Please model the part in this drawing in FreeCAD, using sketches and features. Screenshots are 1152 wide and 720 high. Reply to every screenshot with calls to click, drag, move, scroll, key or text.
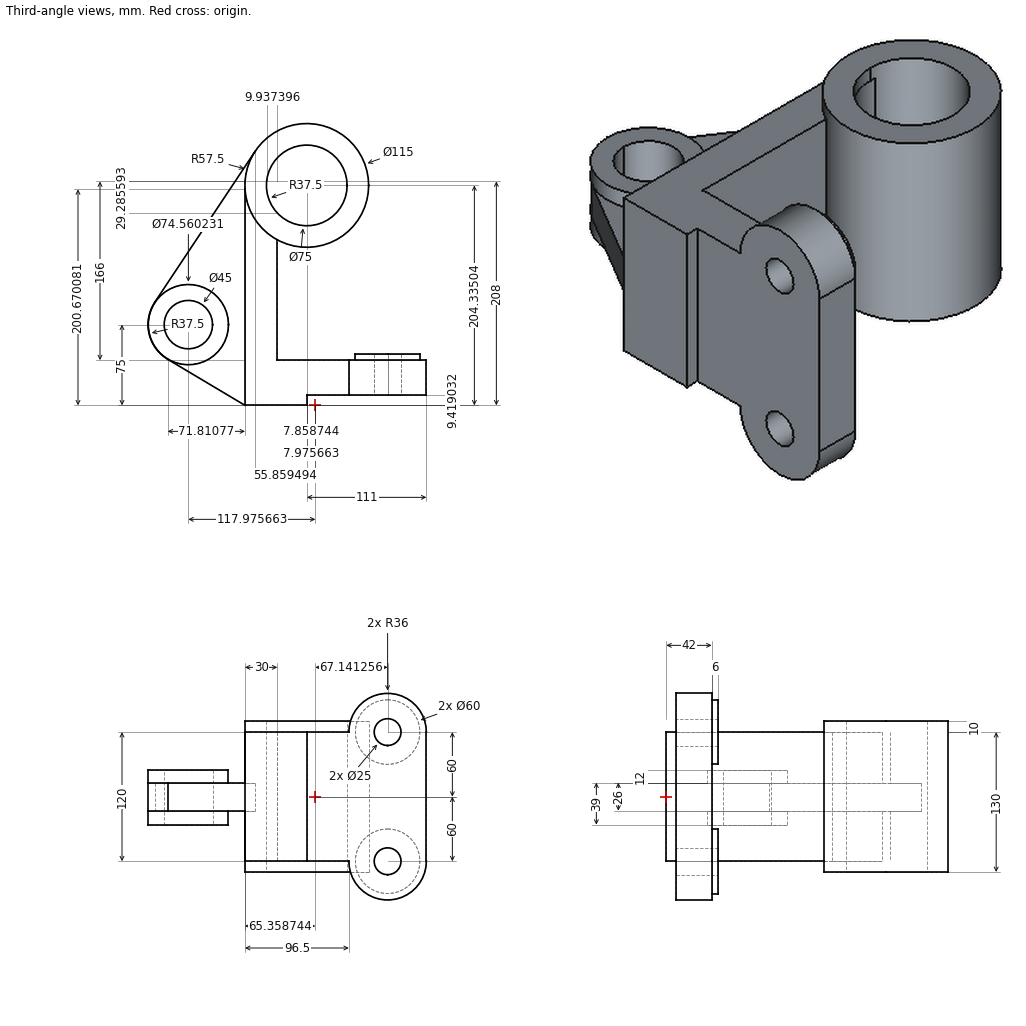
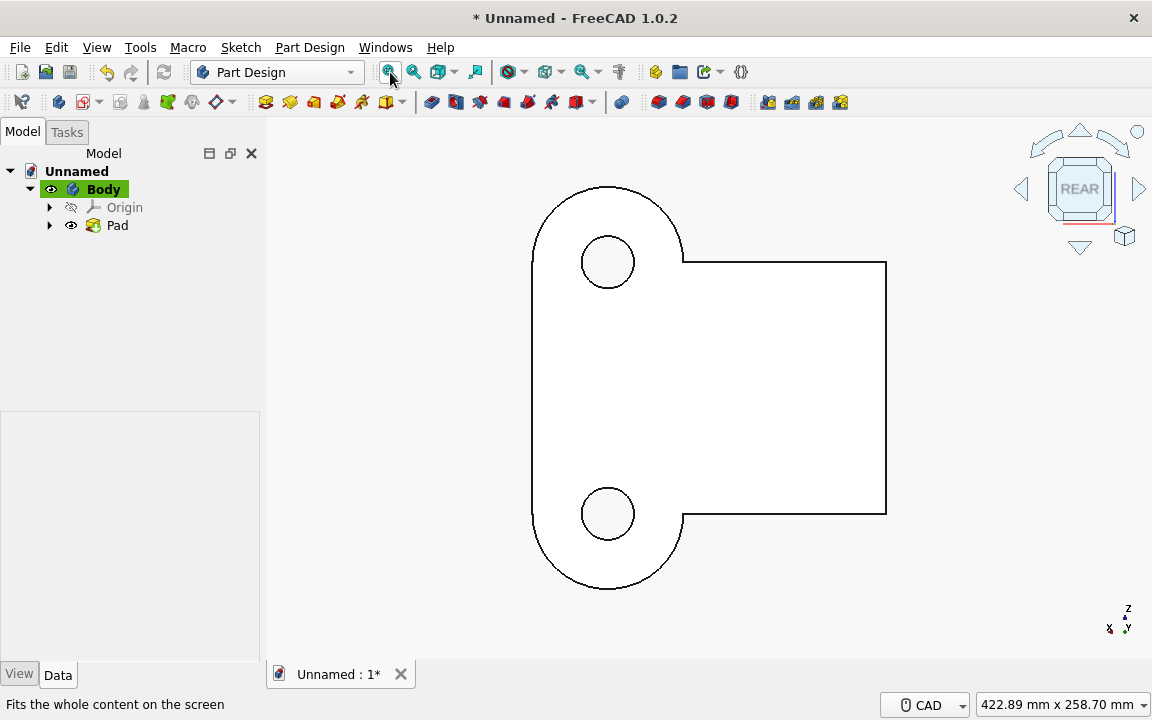
click(709, 387)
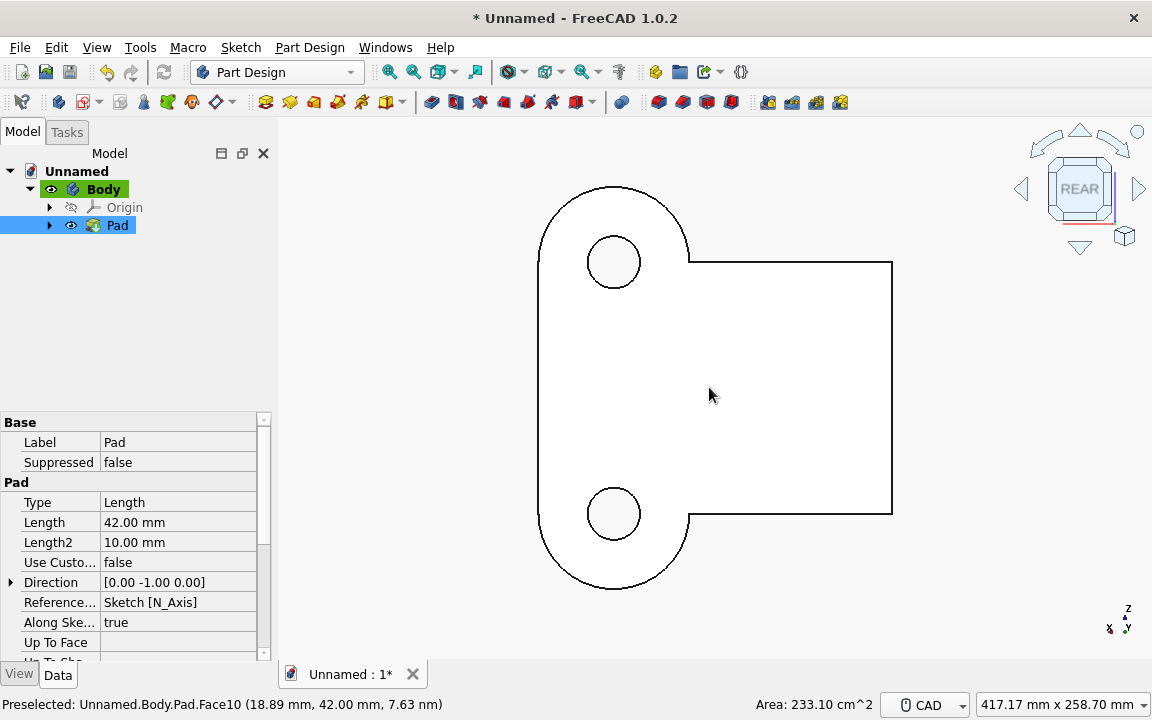
click(84, 102)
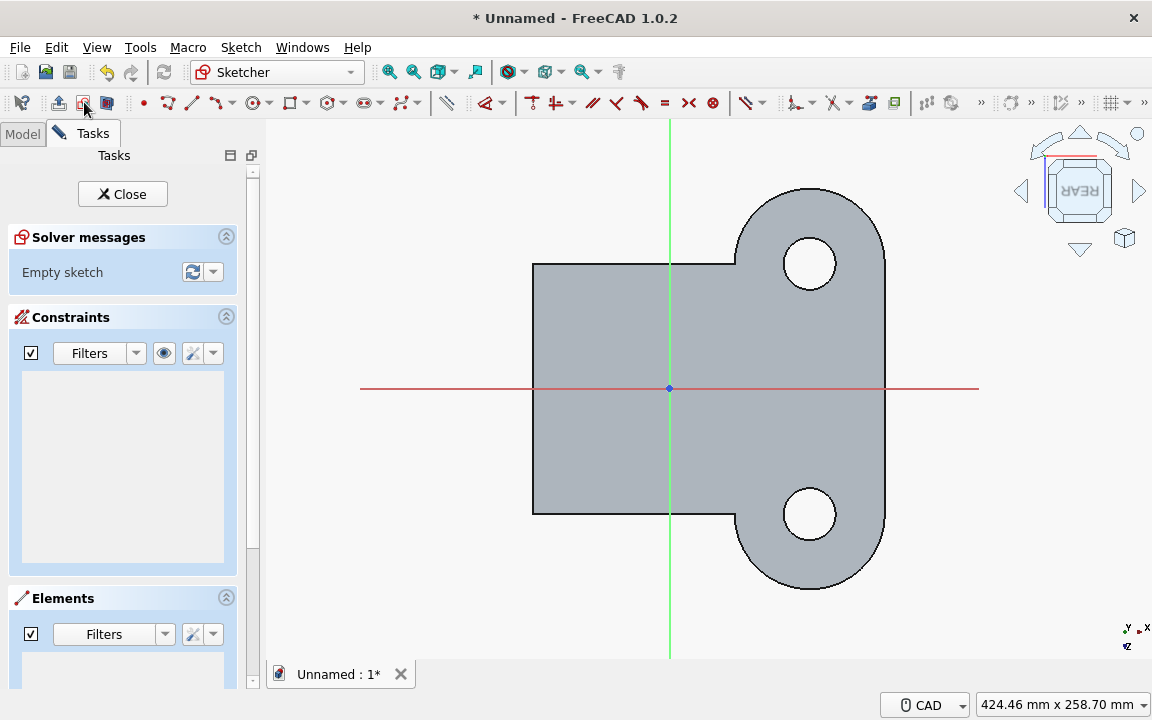
scroll(522, 389, up, 2)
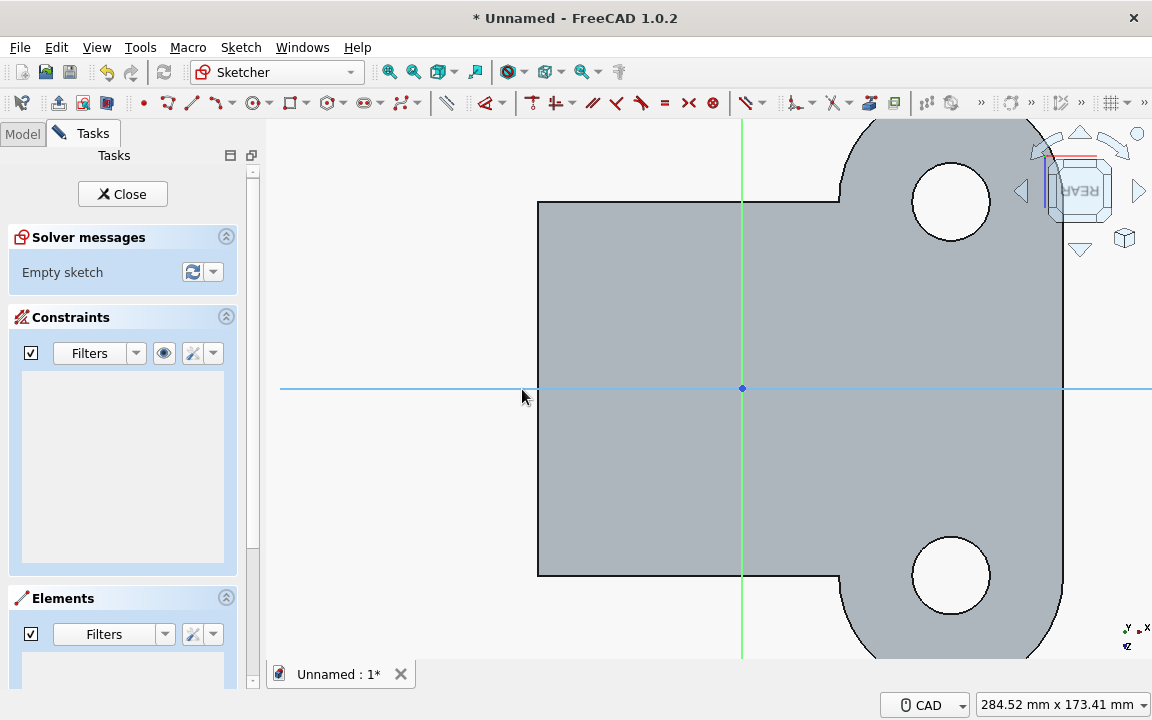
click(290, 104)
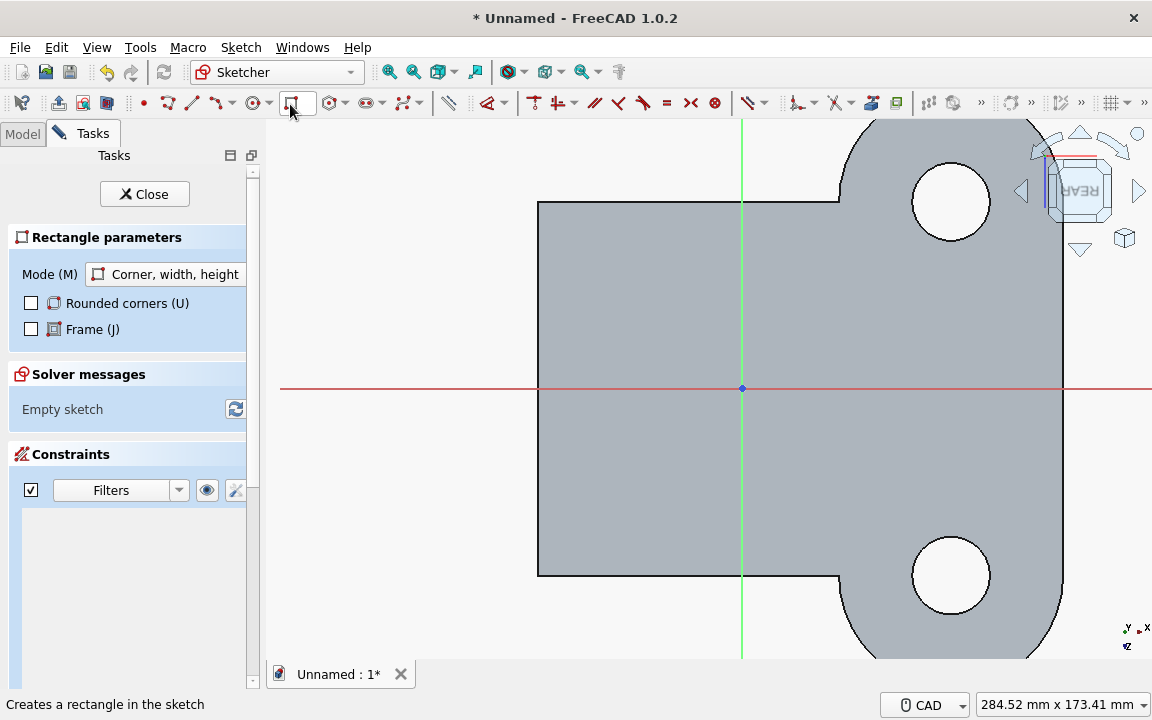
click(538, 202)
move(632, 576)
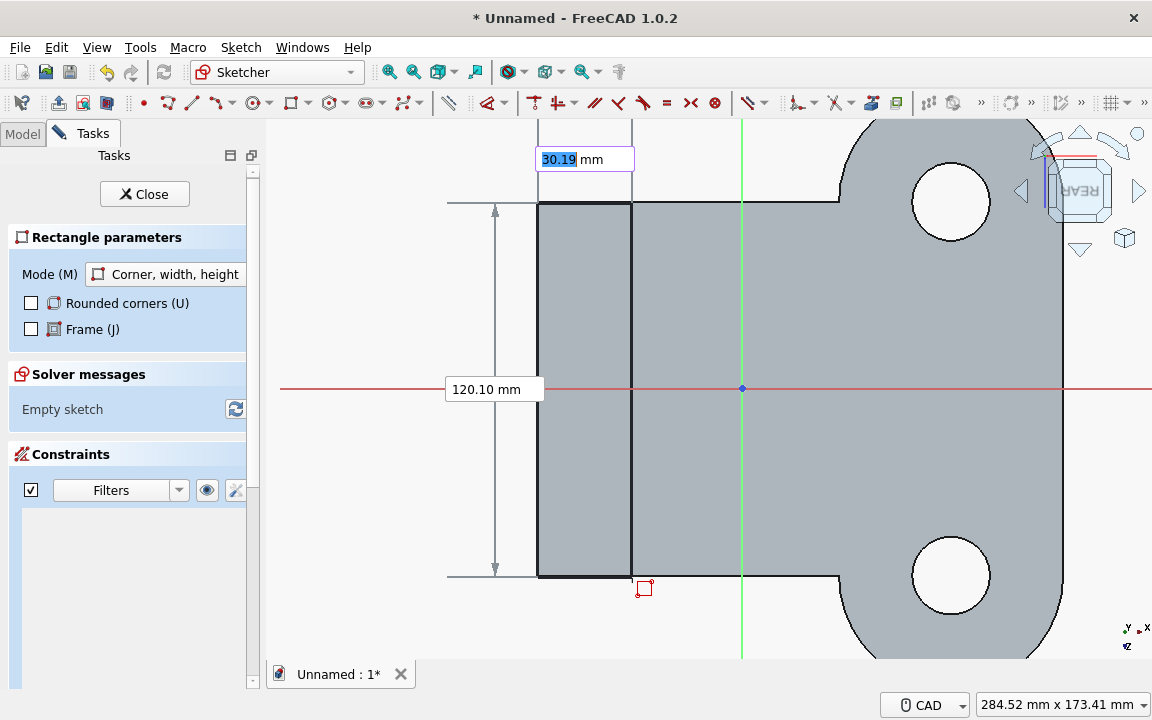
text(30)
key(Tab)
text(120)
key(Return)
key(Escape)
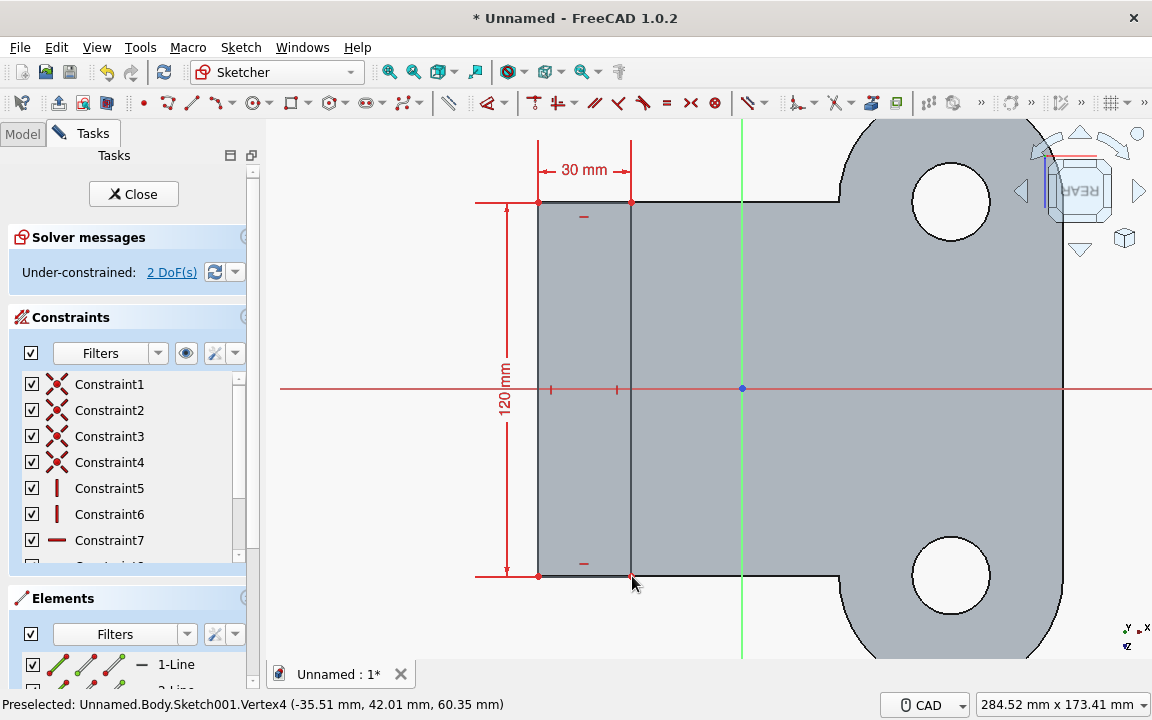
click(488, 104)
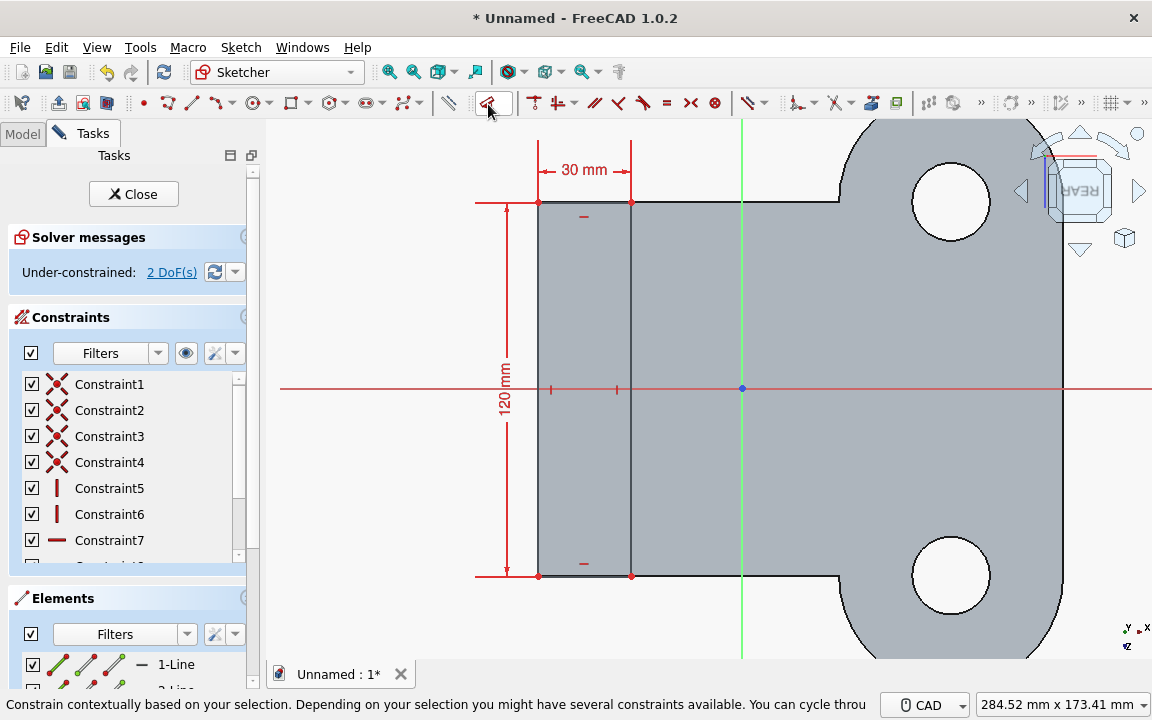
click(538, 203)
click(504, 296)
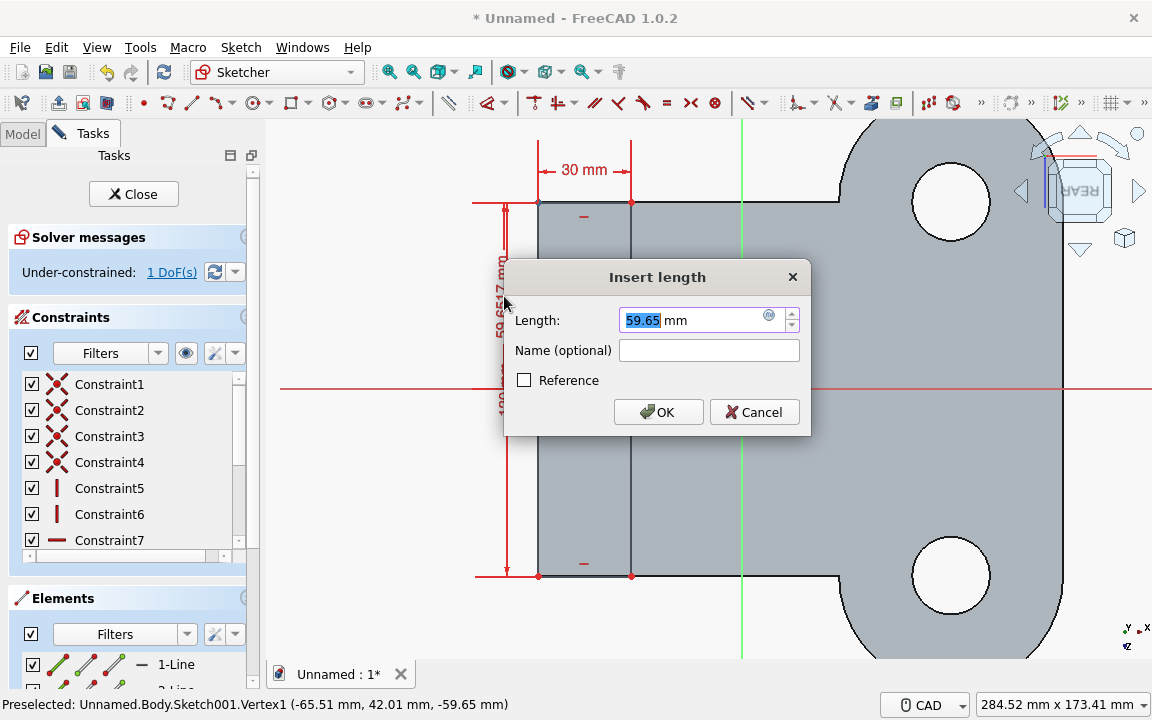
text(60)
key(Return)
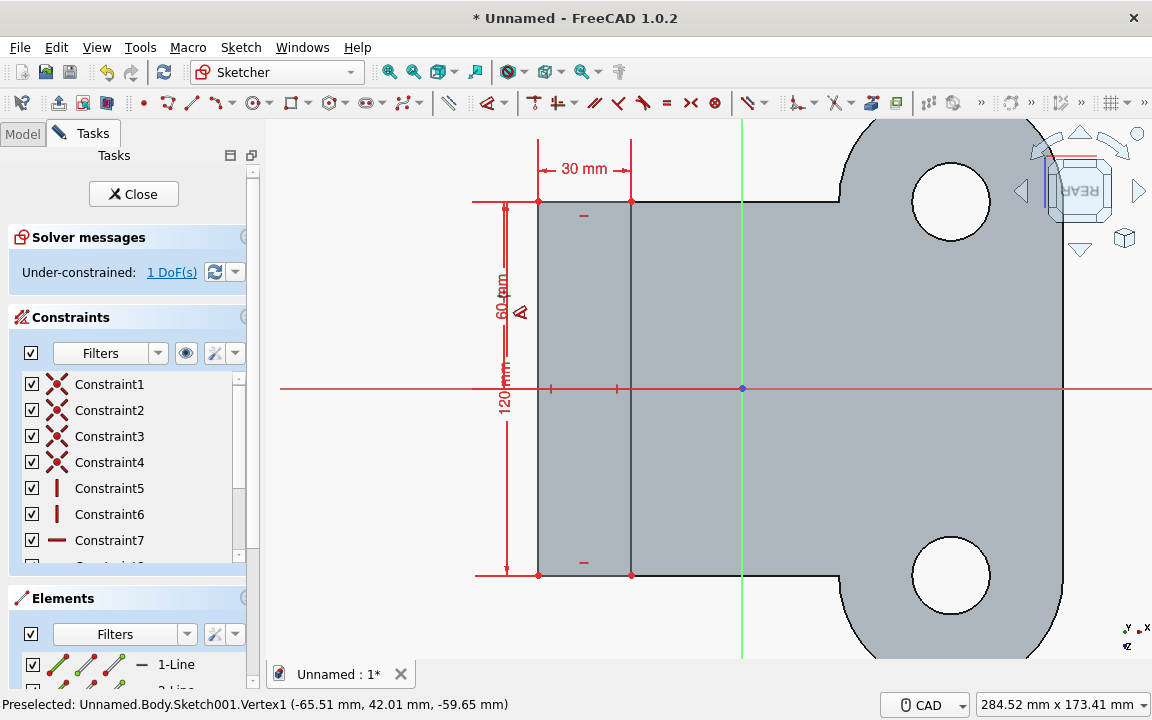
click(538, 202)
click(640, 168)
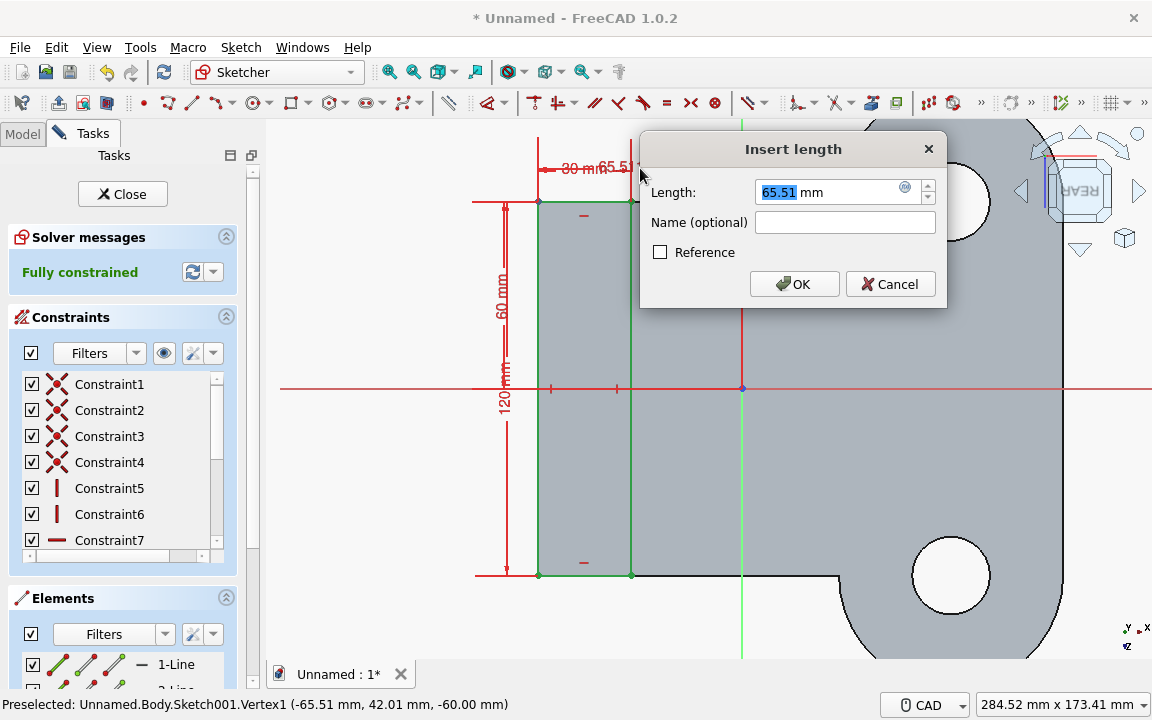
text(65.358744)
key(Return)
key(Escape)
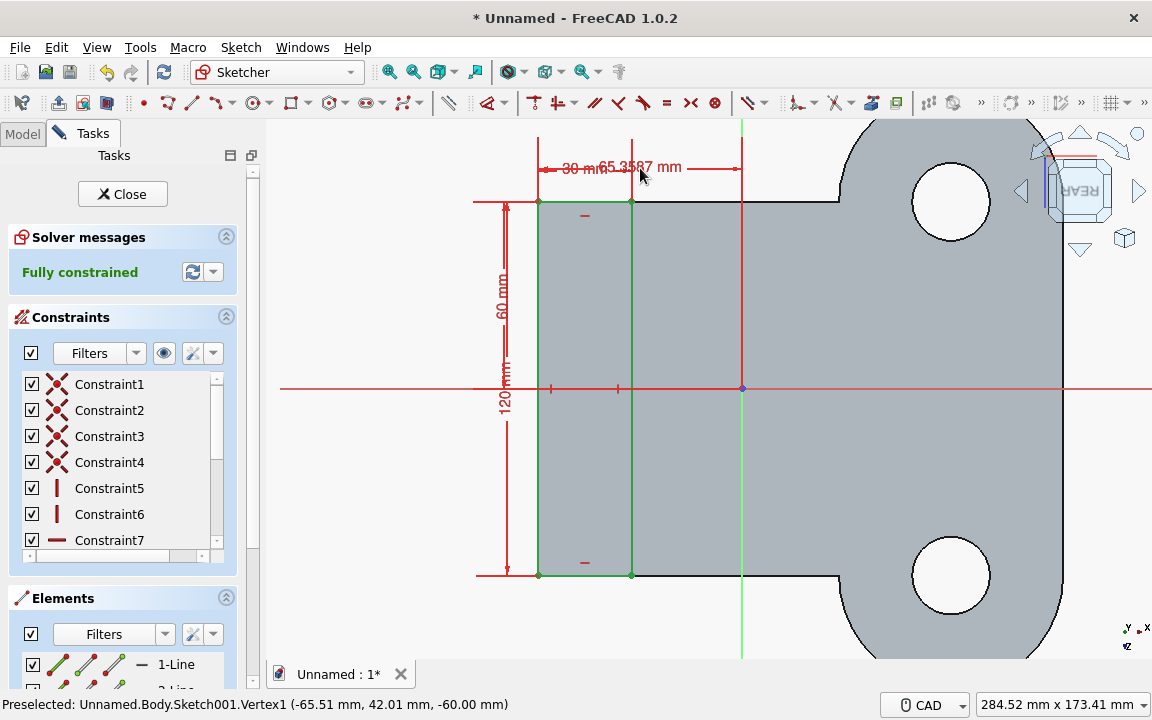
click(123, 194)